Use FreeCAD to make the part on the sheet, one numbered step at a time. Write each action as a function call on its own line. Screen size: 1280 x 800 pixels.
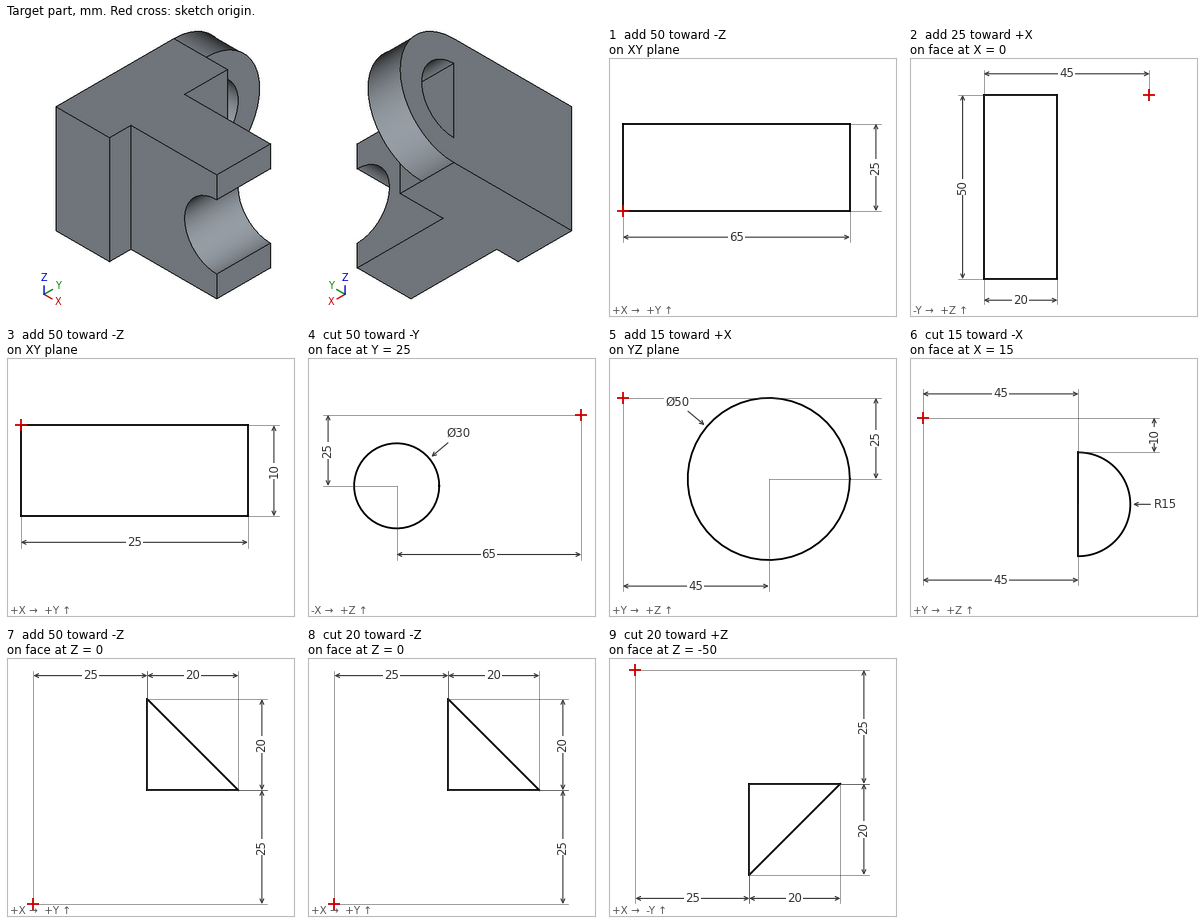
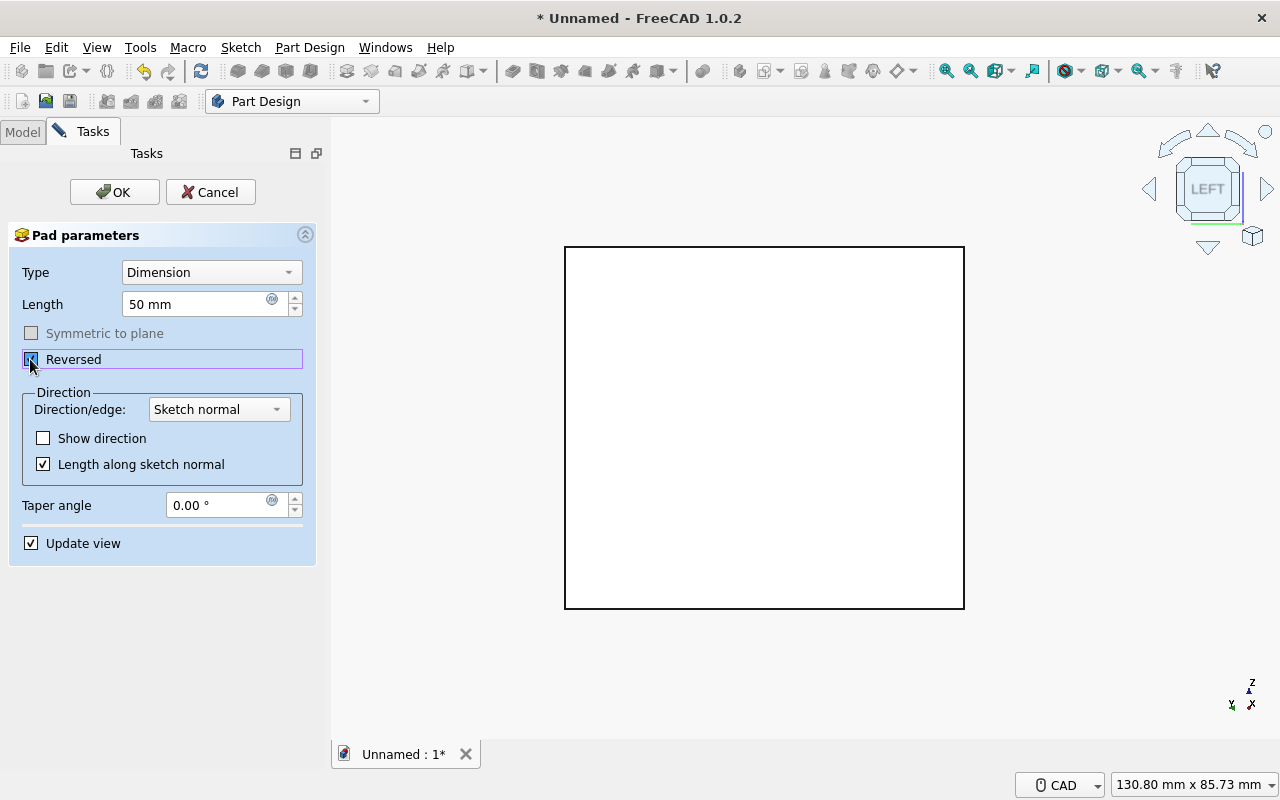
click(115, 192)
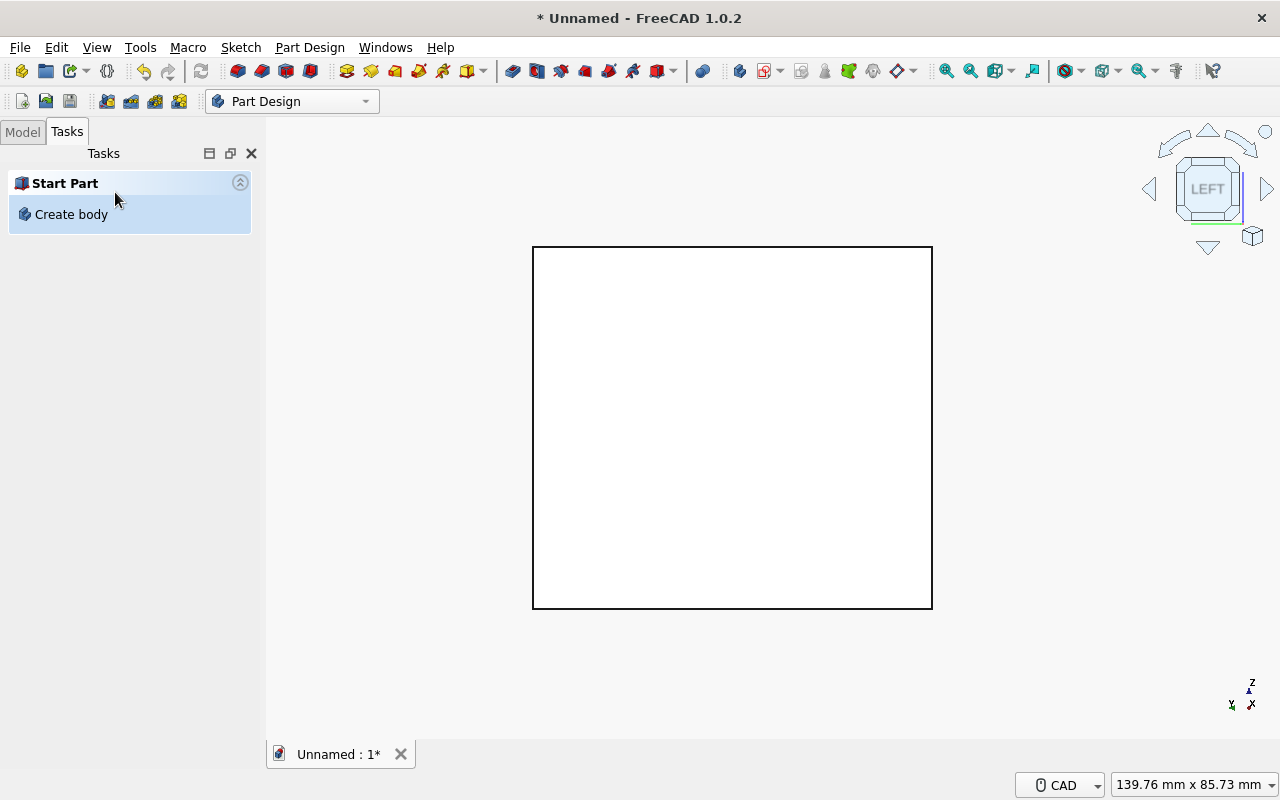
key(4)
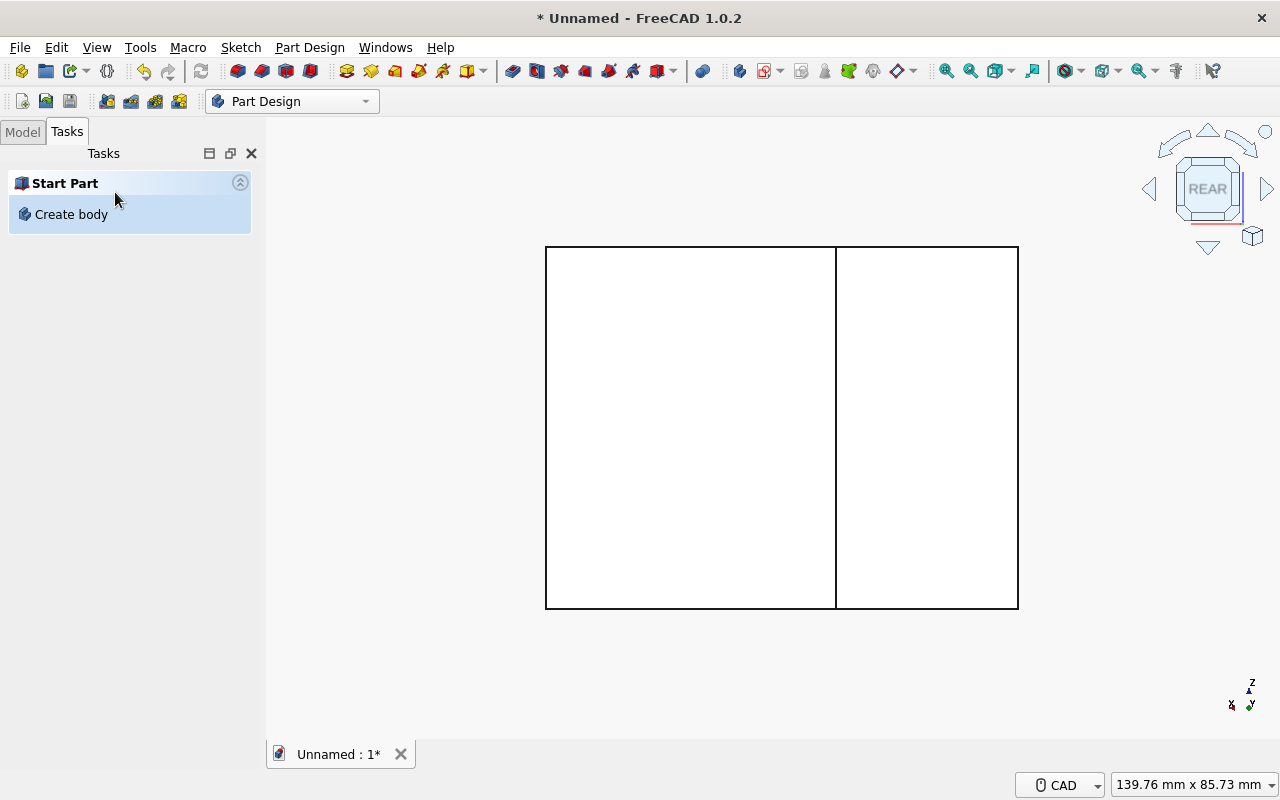
click(691, 427)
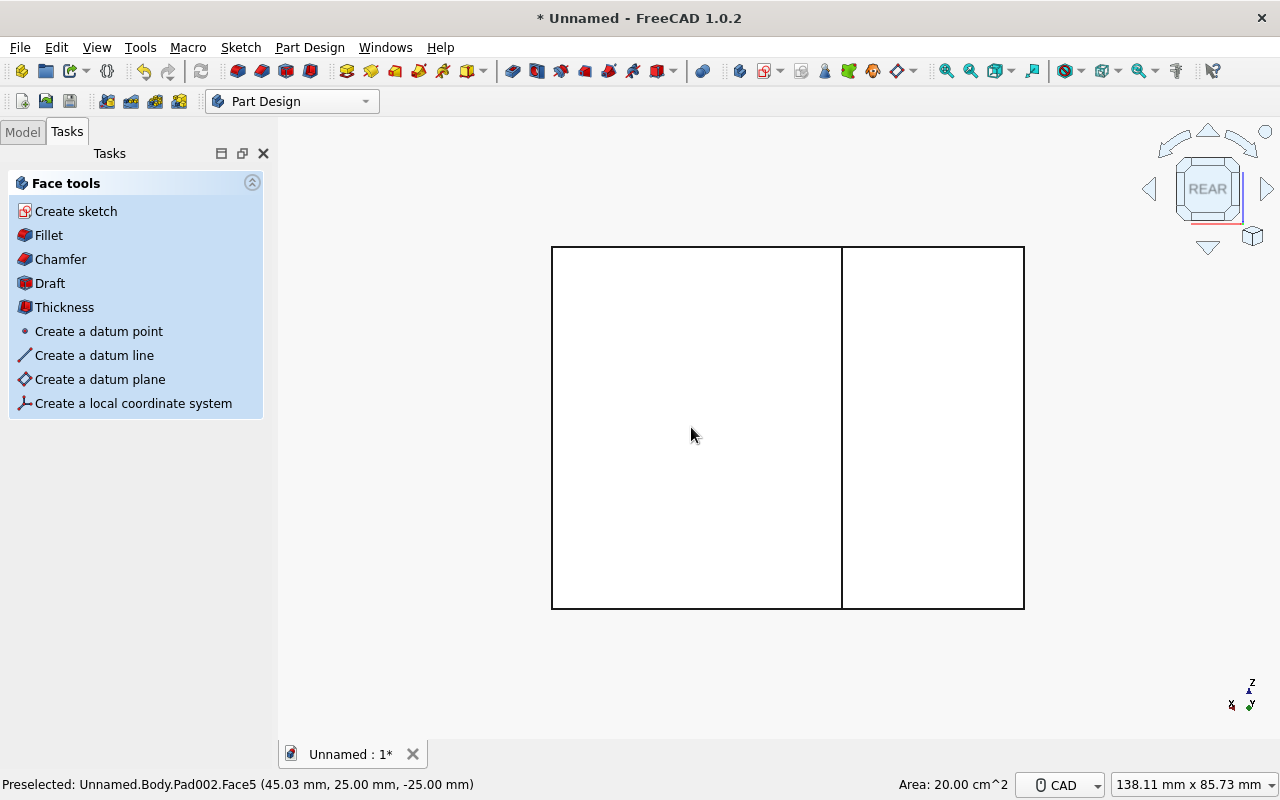
click(764, 72)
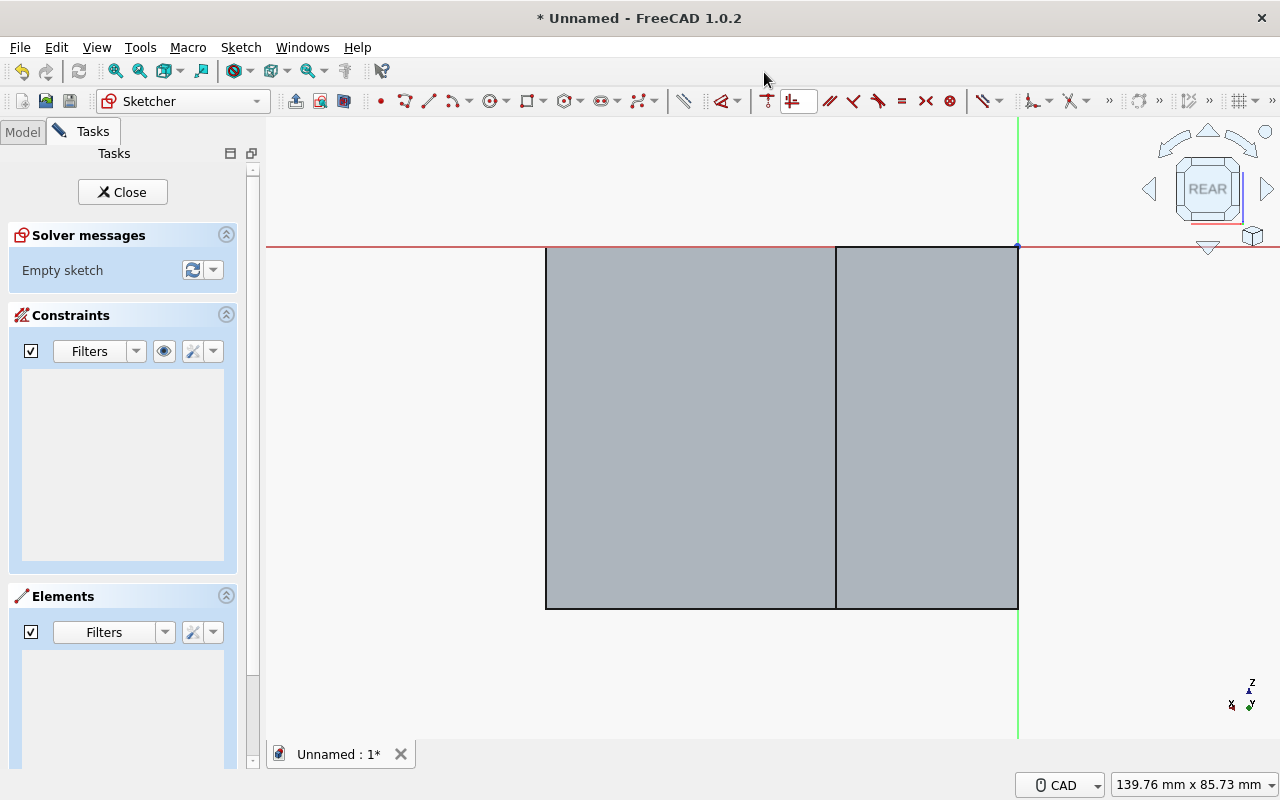
scroll(353, 428, up, 3)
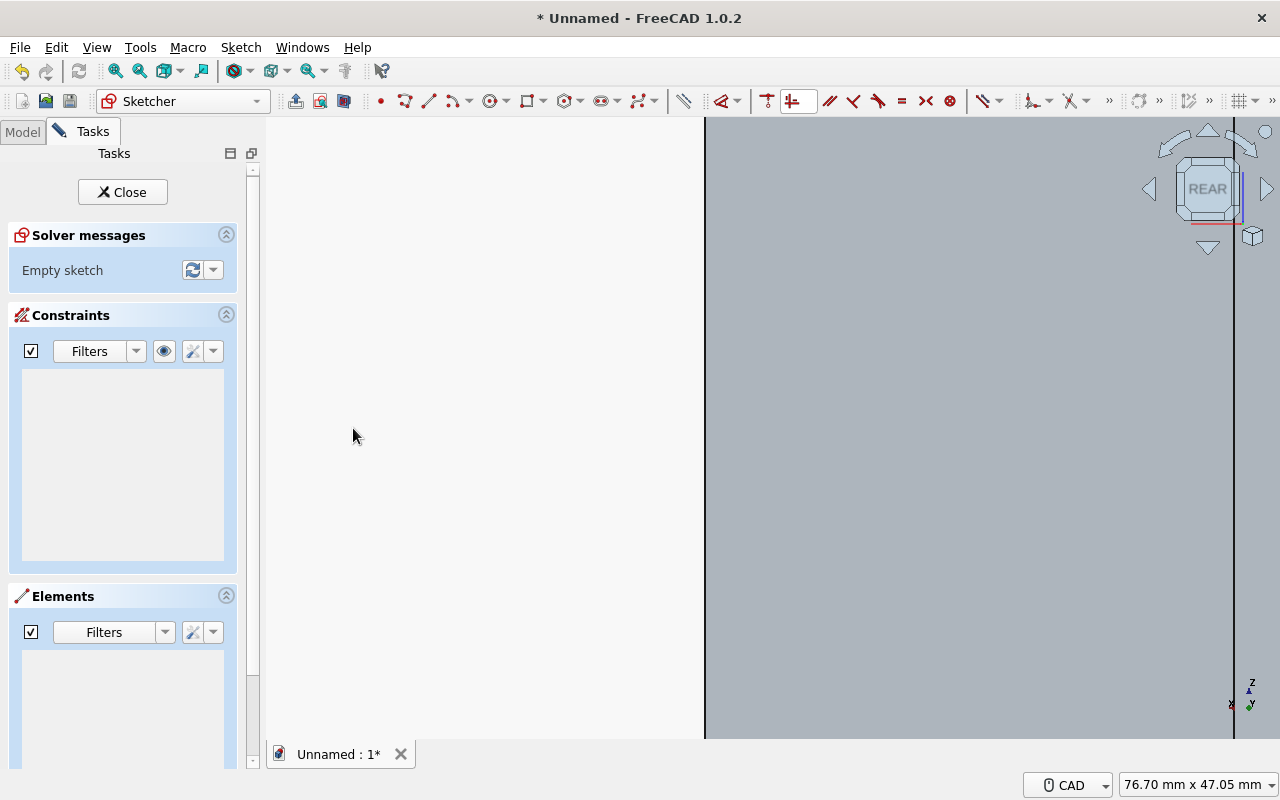
click(490, 102)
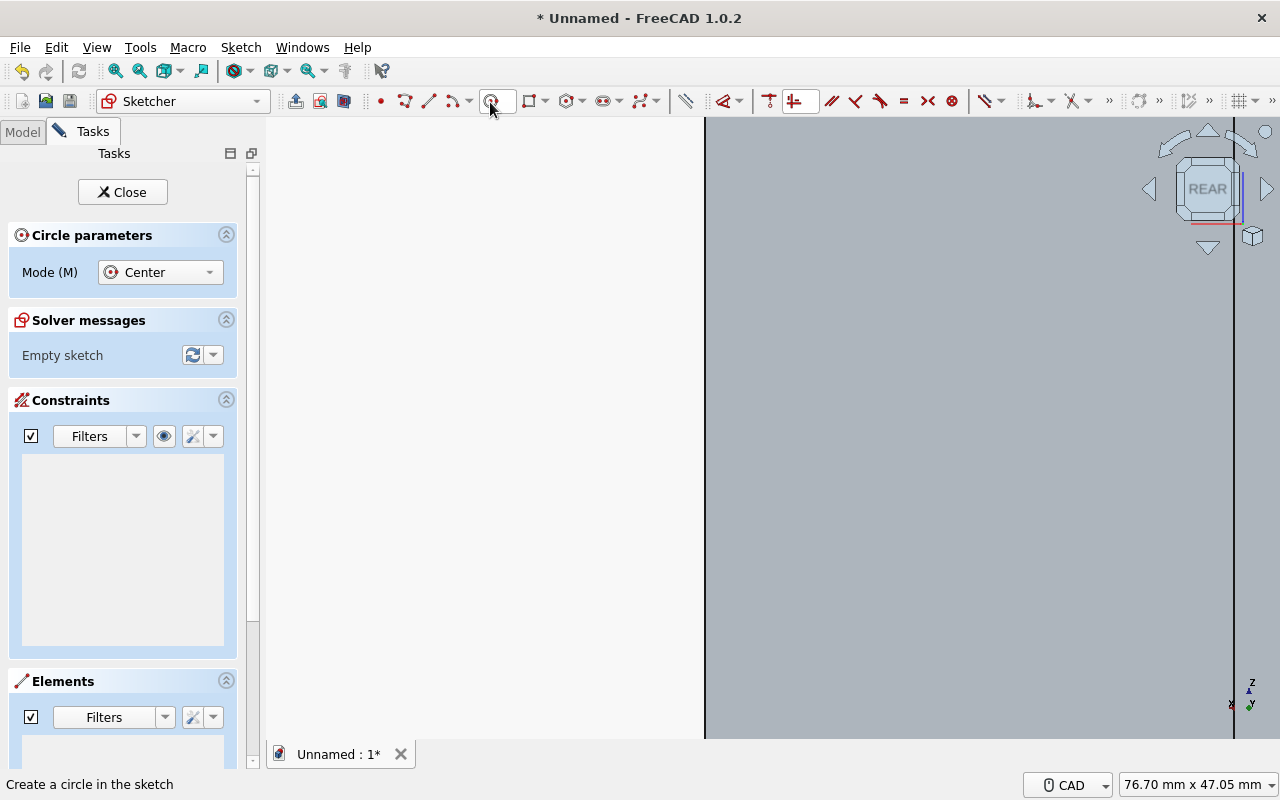
click(705, 428)
move(845, 287)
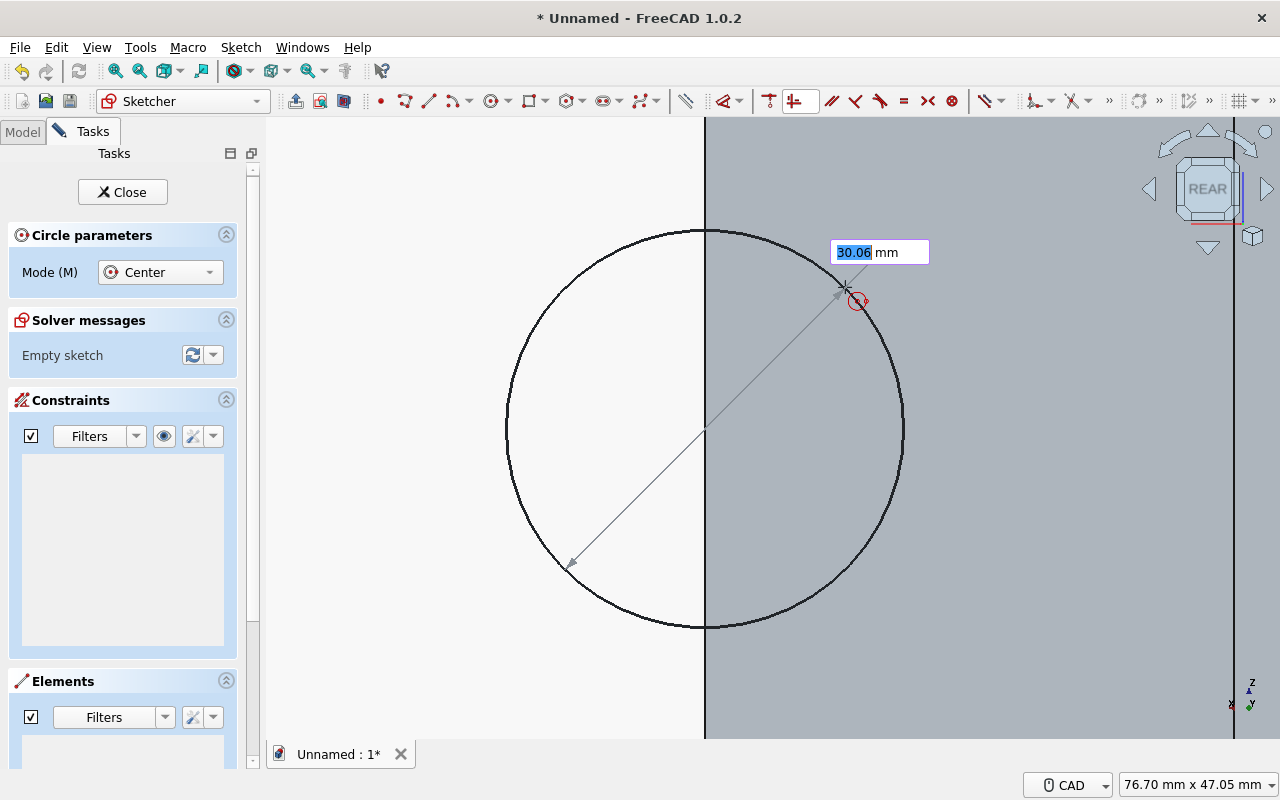
text(30)
key(Return)
key(Escape)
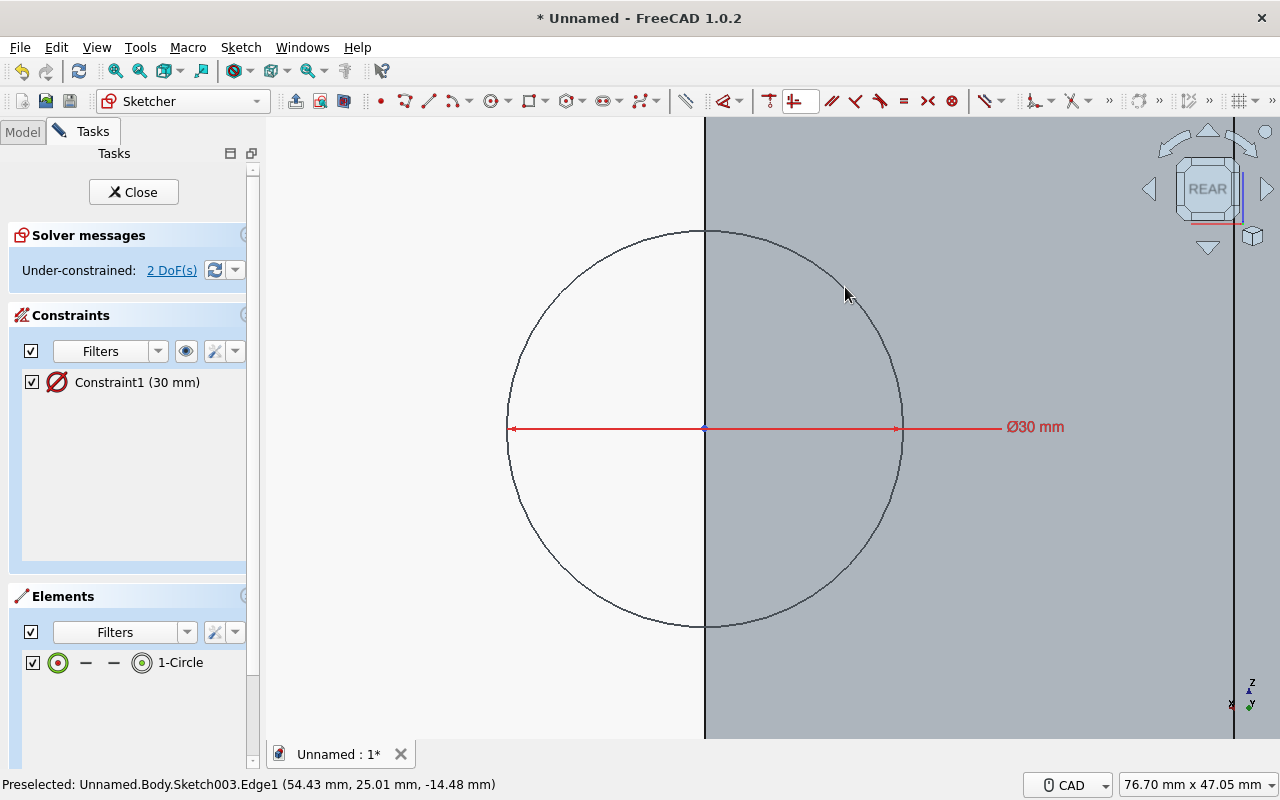
click(705, 429)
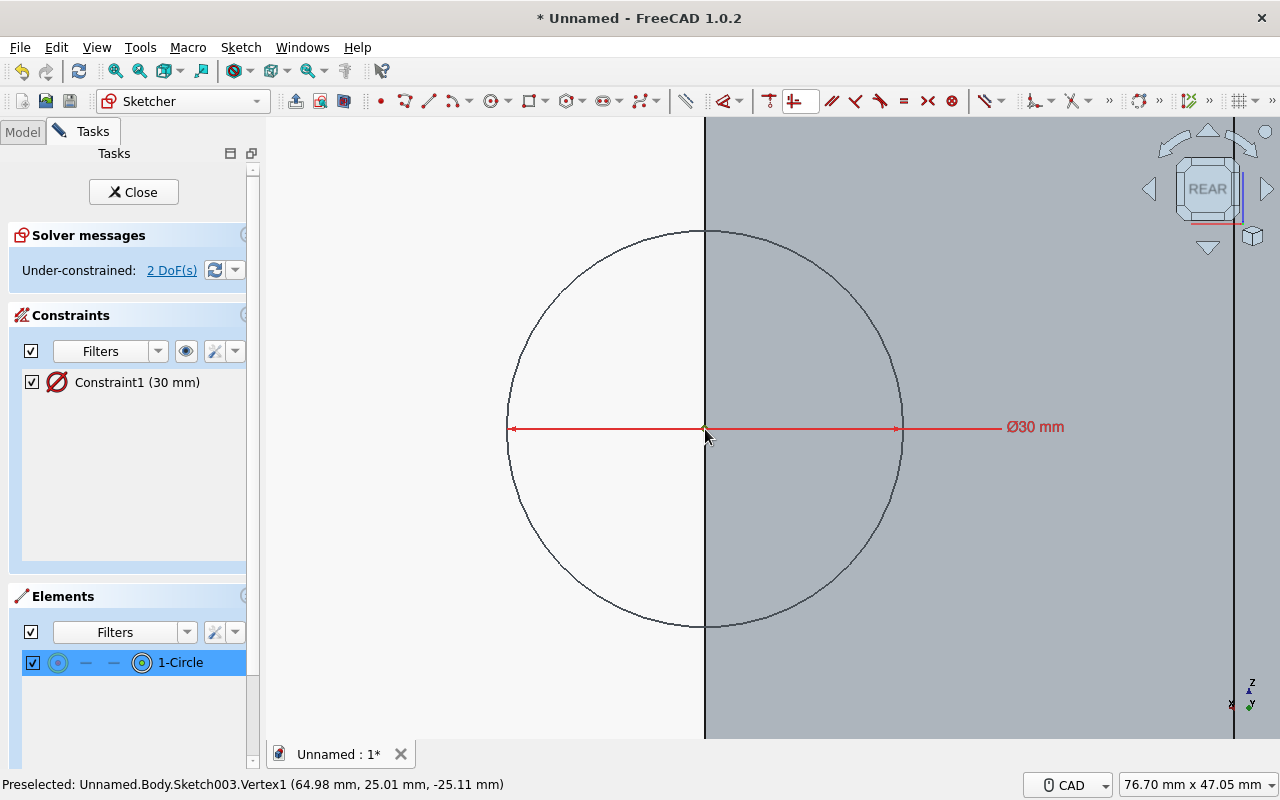
key(l)